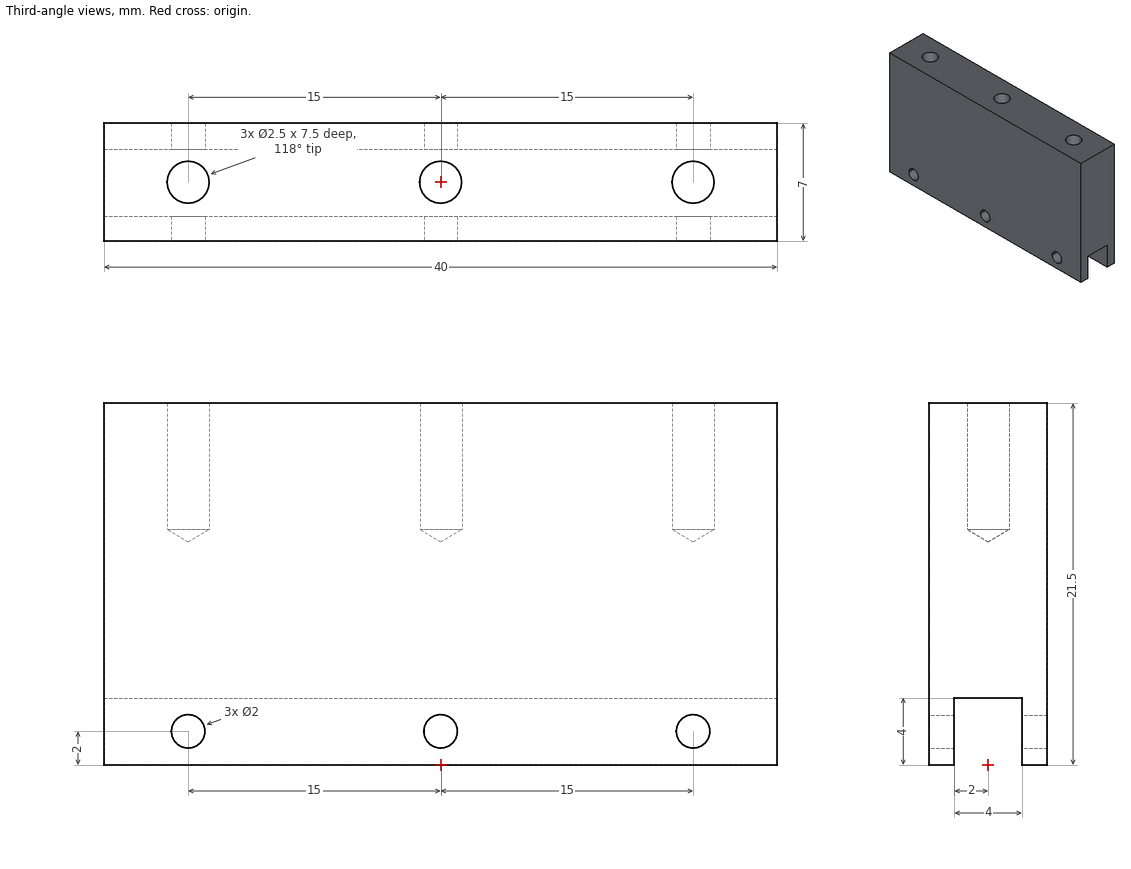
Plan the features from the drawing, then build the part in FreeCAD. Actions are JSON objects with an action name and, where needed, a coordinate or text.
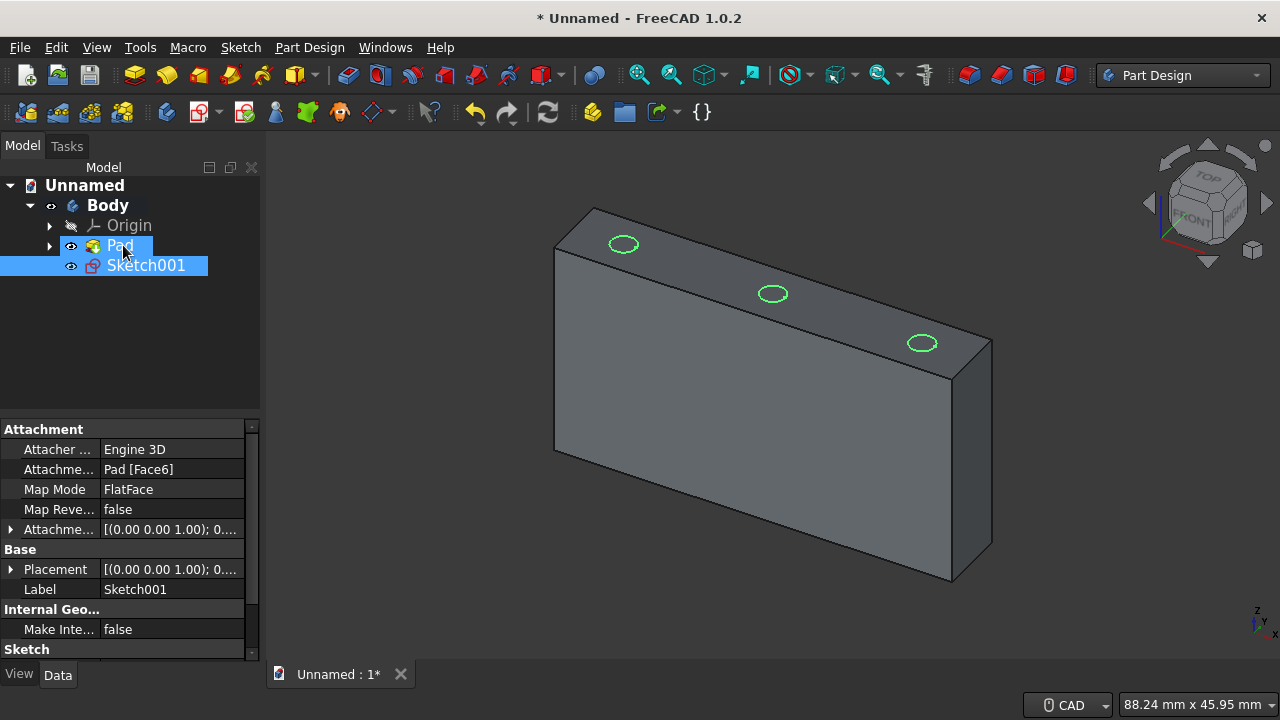
{"action": "left_click", "coordinate": [382, 76]}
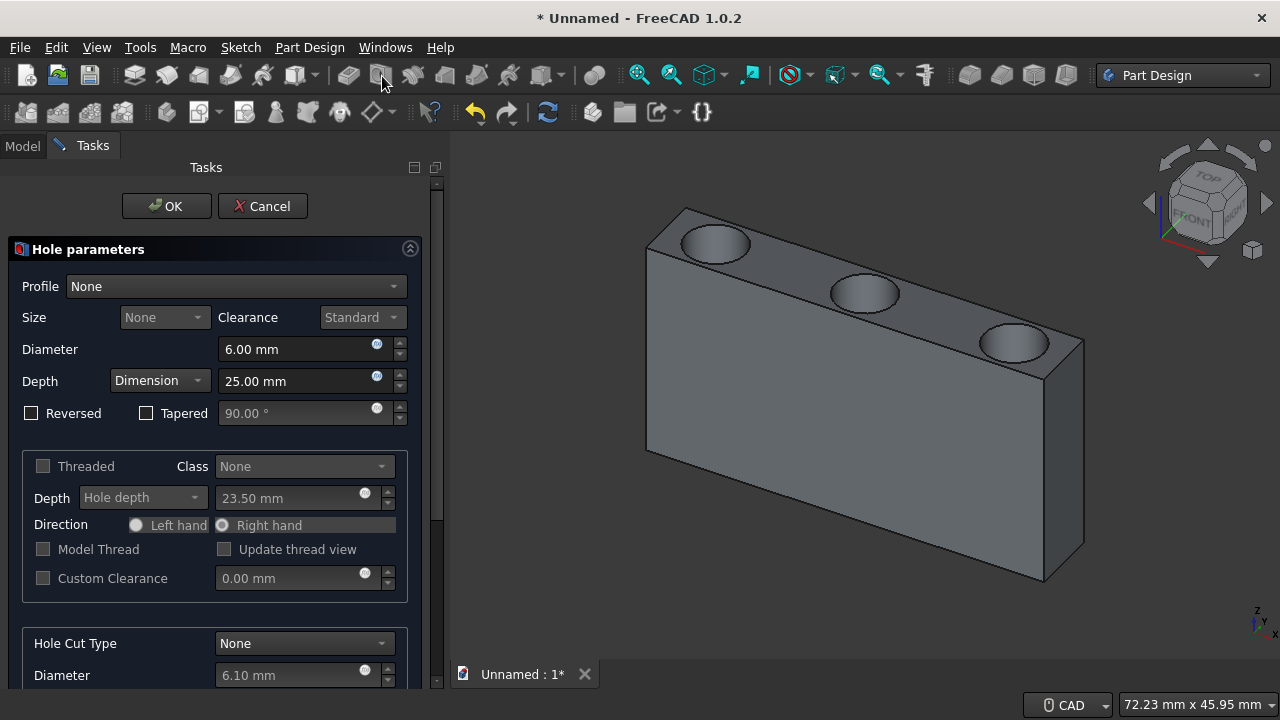
{"action": "triple_click", "coordinate": [305, 349]}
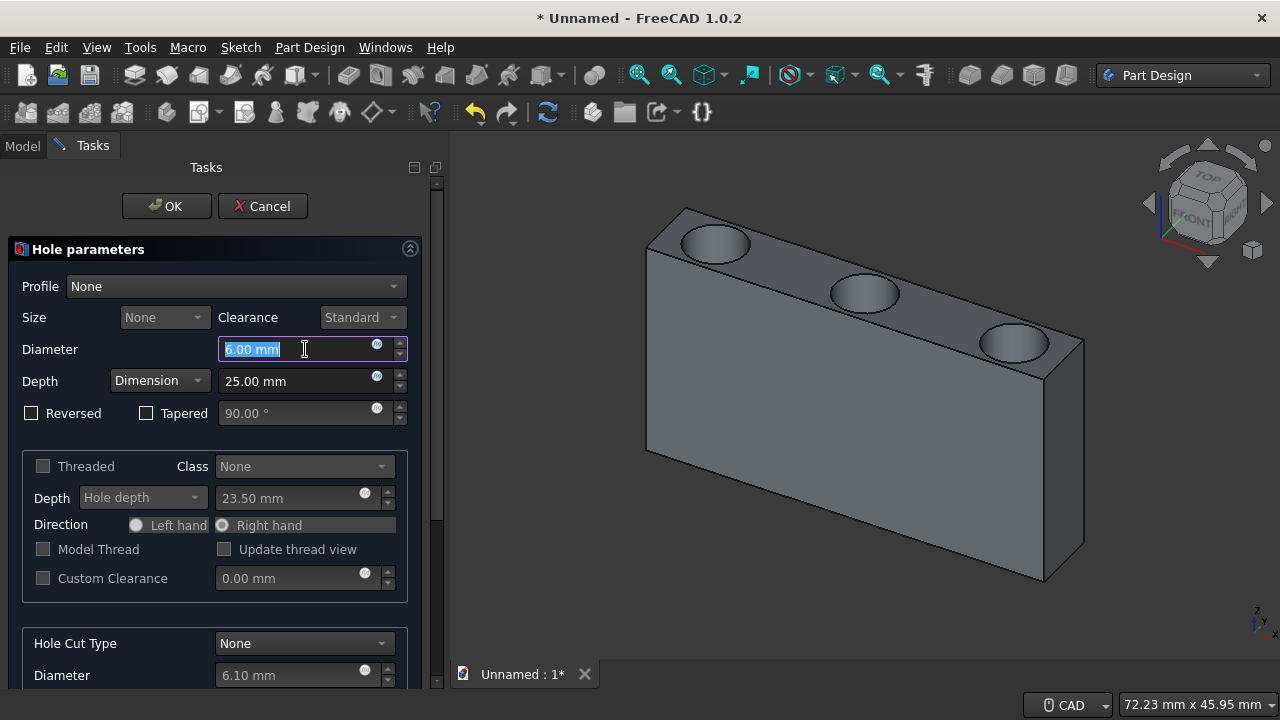
{"action": "type", "text": "2.5"}
{"action": "key", "text": "Tab"}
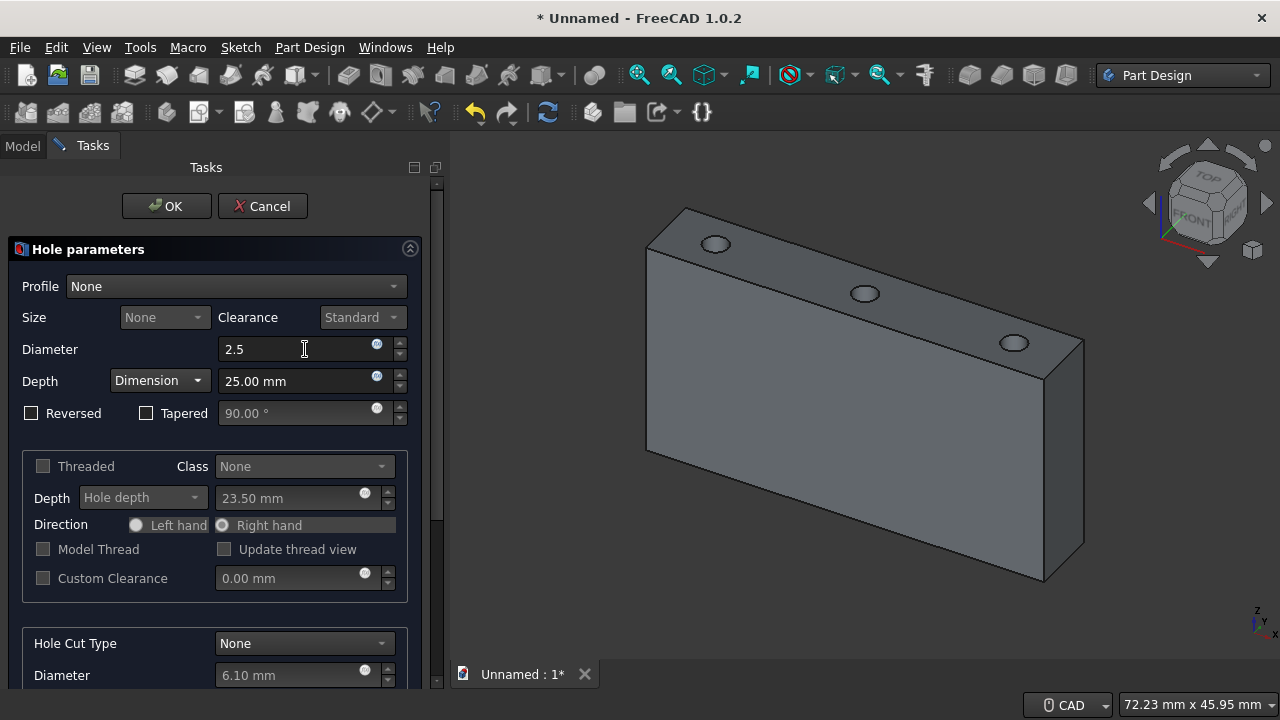
{"action": "triple_click", "coordinate": [305, 381]}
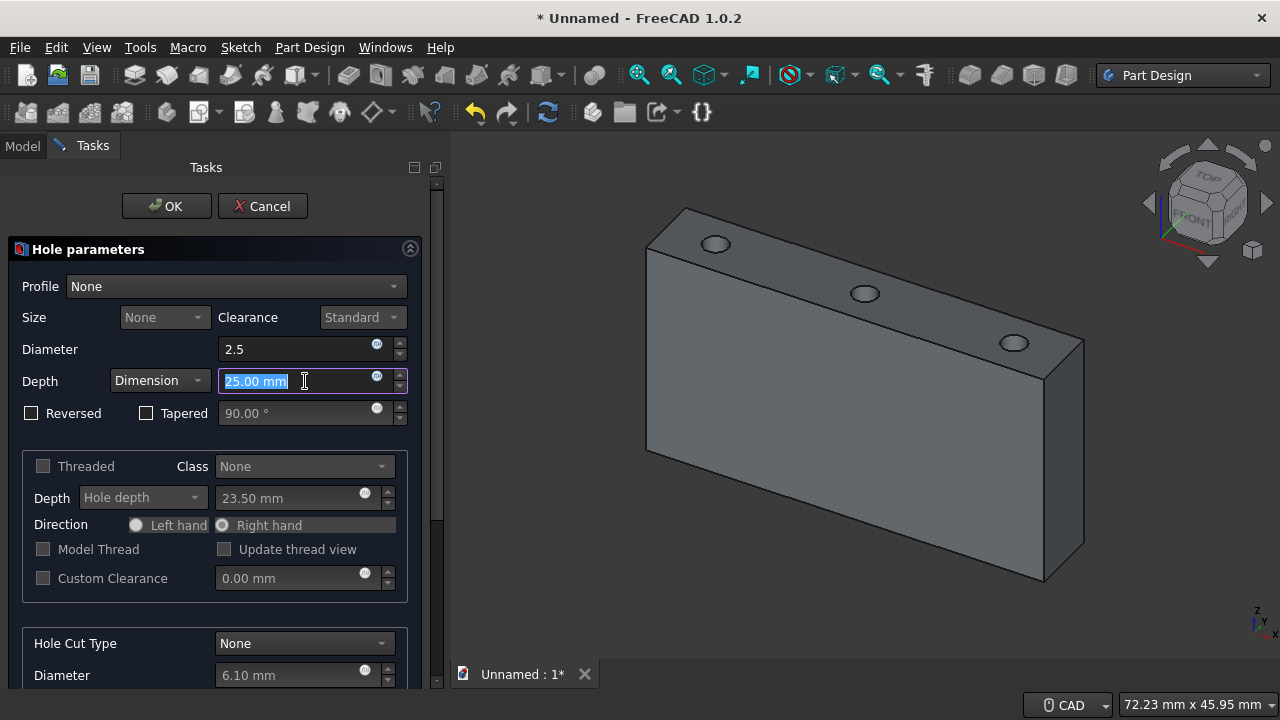
{"action": "type", "text": "7.5"}
{"action": "key", "text": "Tab"}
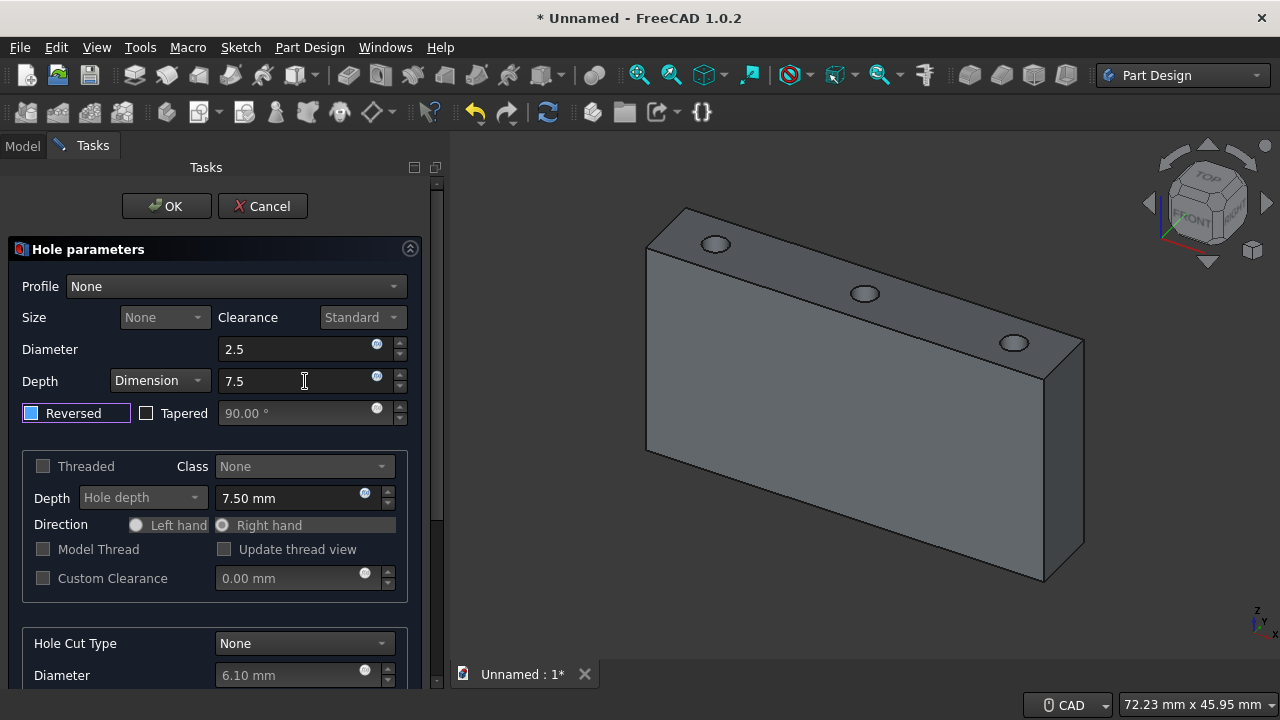
{"action": "left_click", "coordinate": [167, 206]}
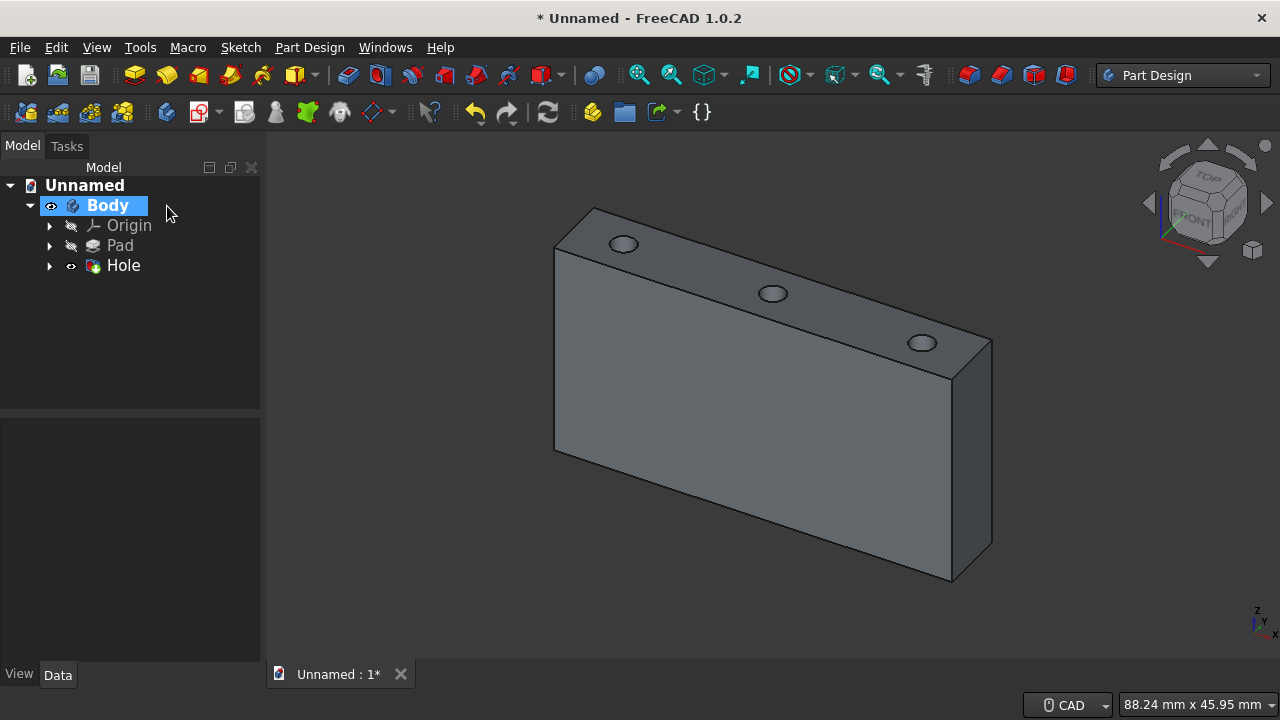
{"action": "left_click", "coordinate": [972, 402]}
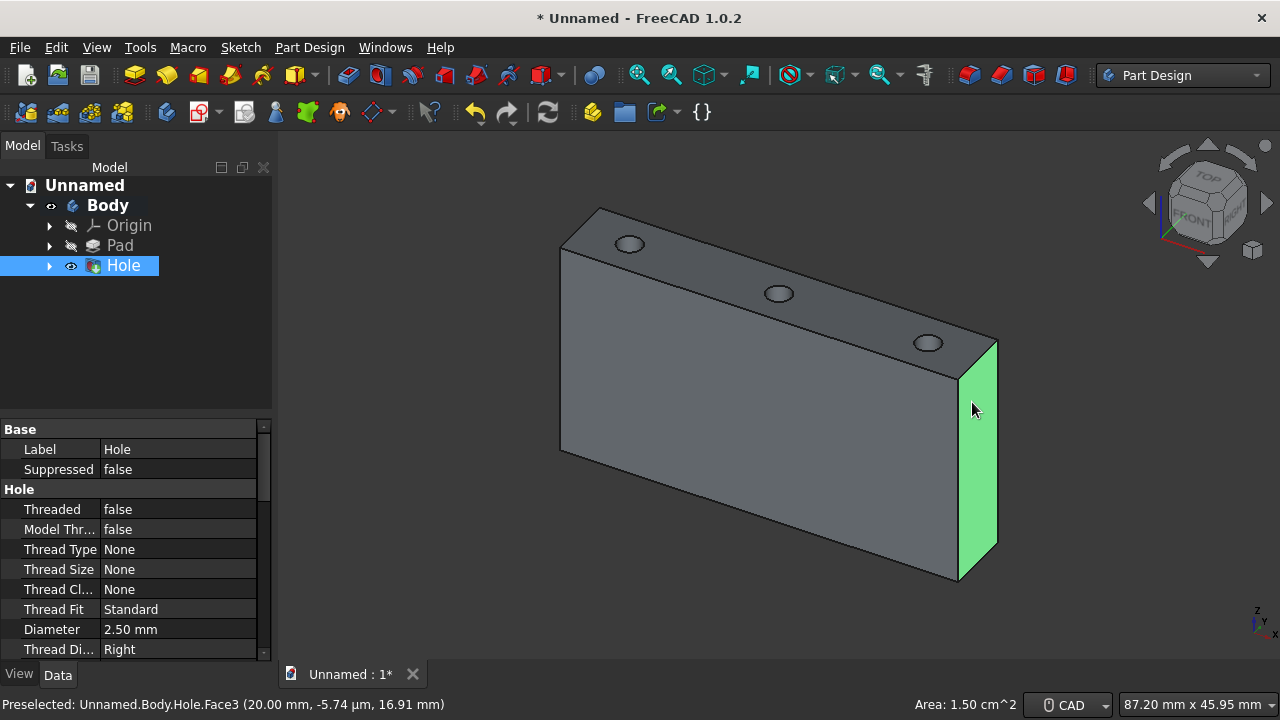
{"action": "left_click", "coordinate": [200, 112]}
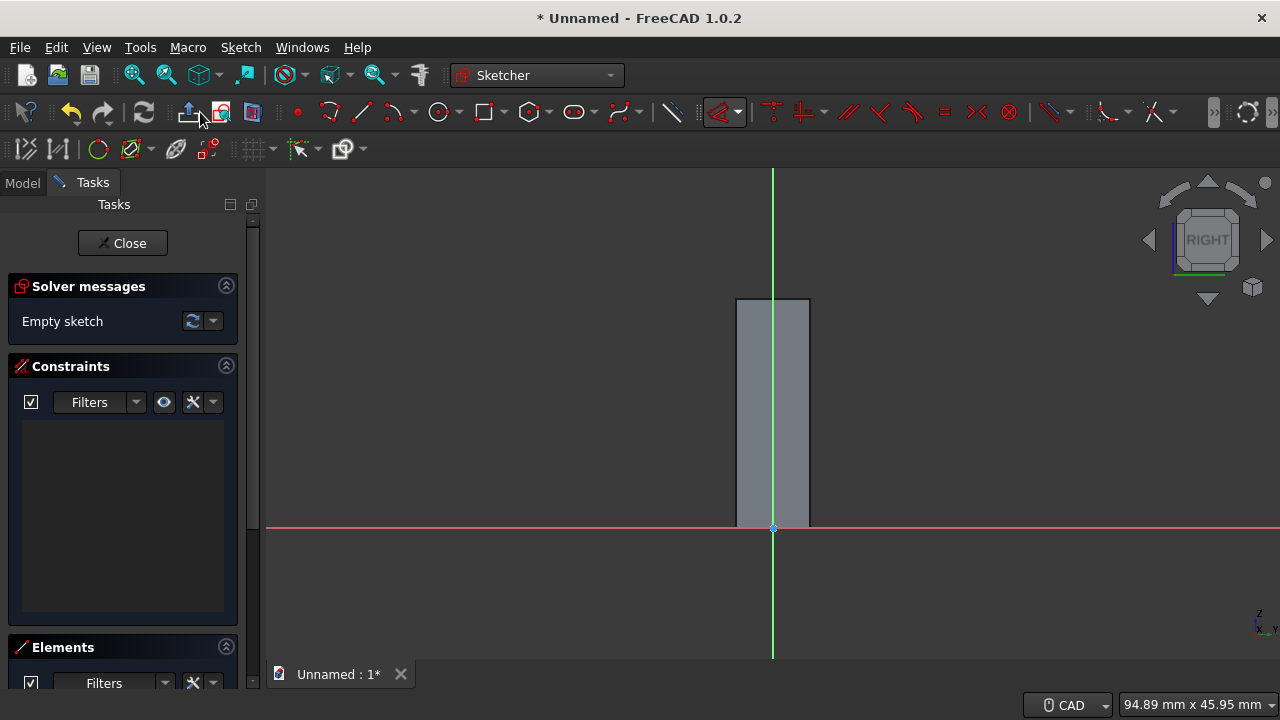
{"action": "scroll", "coordinate": [784, 522], "scroll_direction": "up", "scroll_amount": 10}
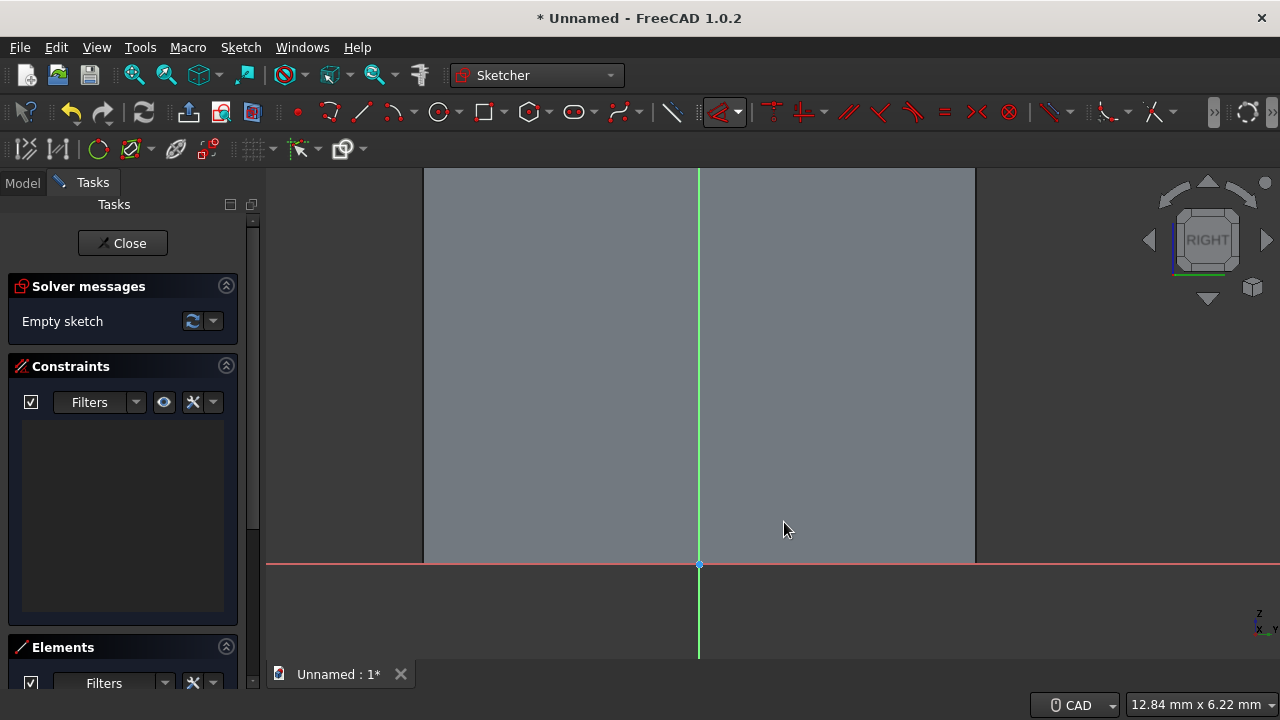
{"action": "left_click", "coordinate": [484, 112]}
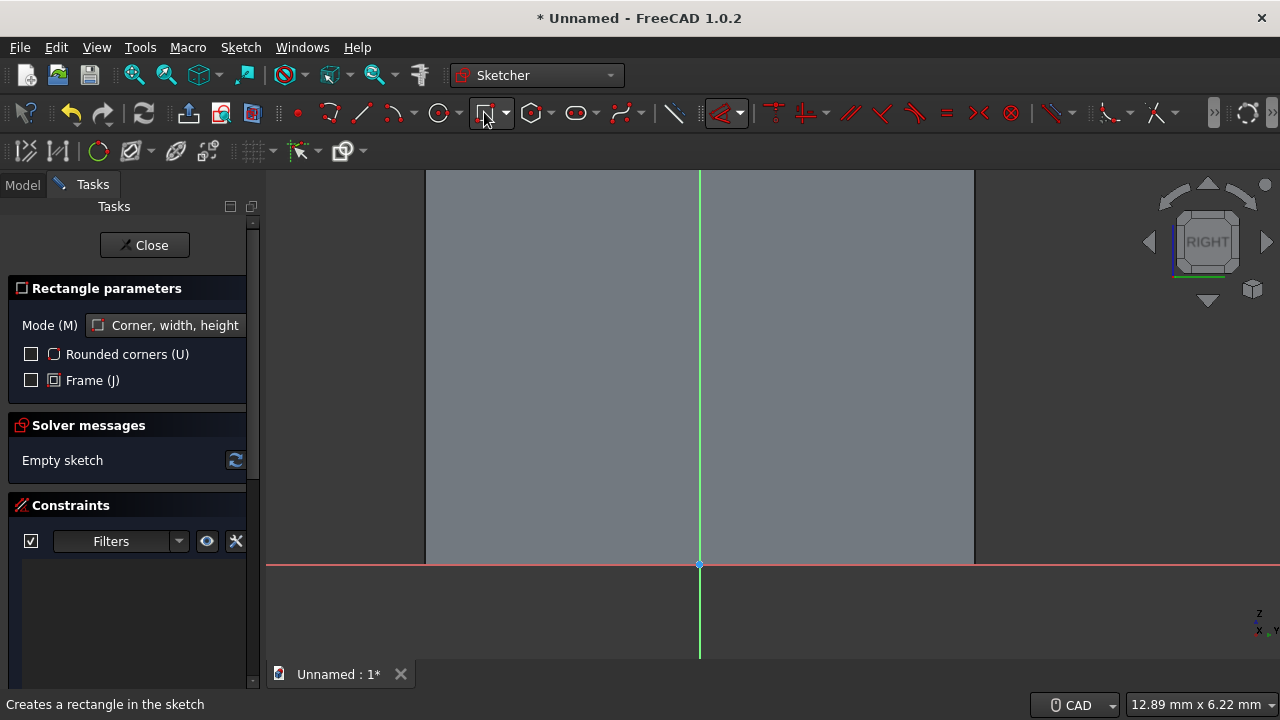
{"action": "left_click", "coordinate": [542, 250]}
{"action": "left_click", "coordinate": [857, 565]}
{"action": "key", "text": "Escape"}